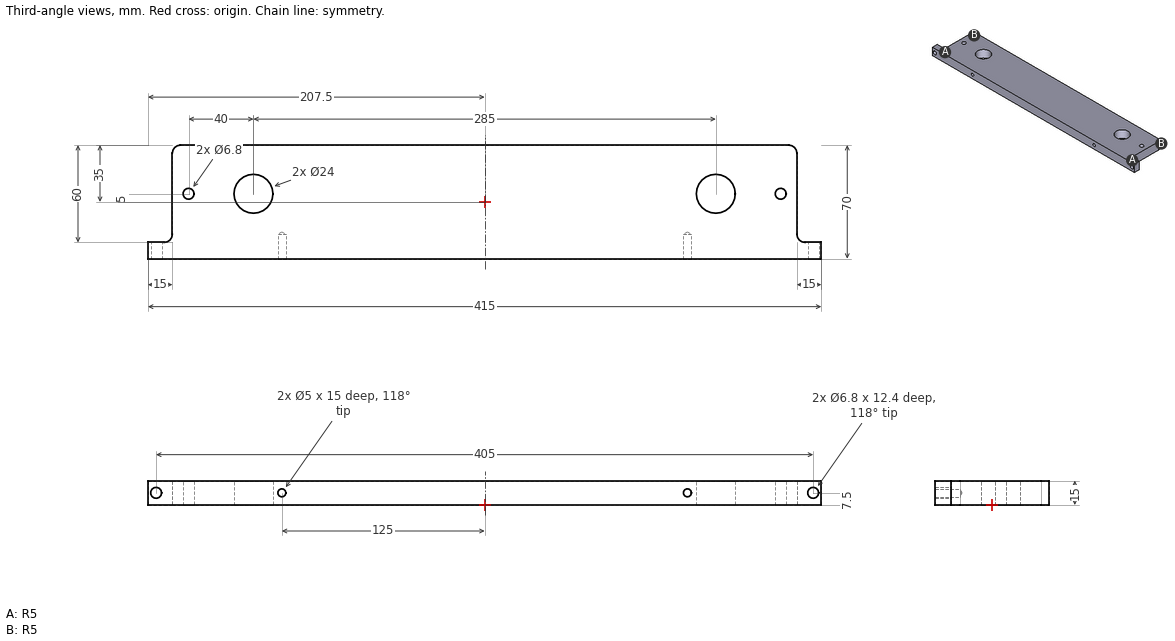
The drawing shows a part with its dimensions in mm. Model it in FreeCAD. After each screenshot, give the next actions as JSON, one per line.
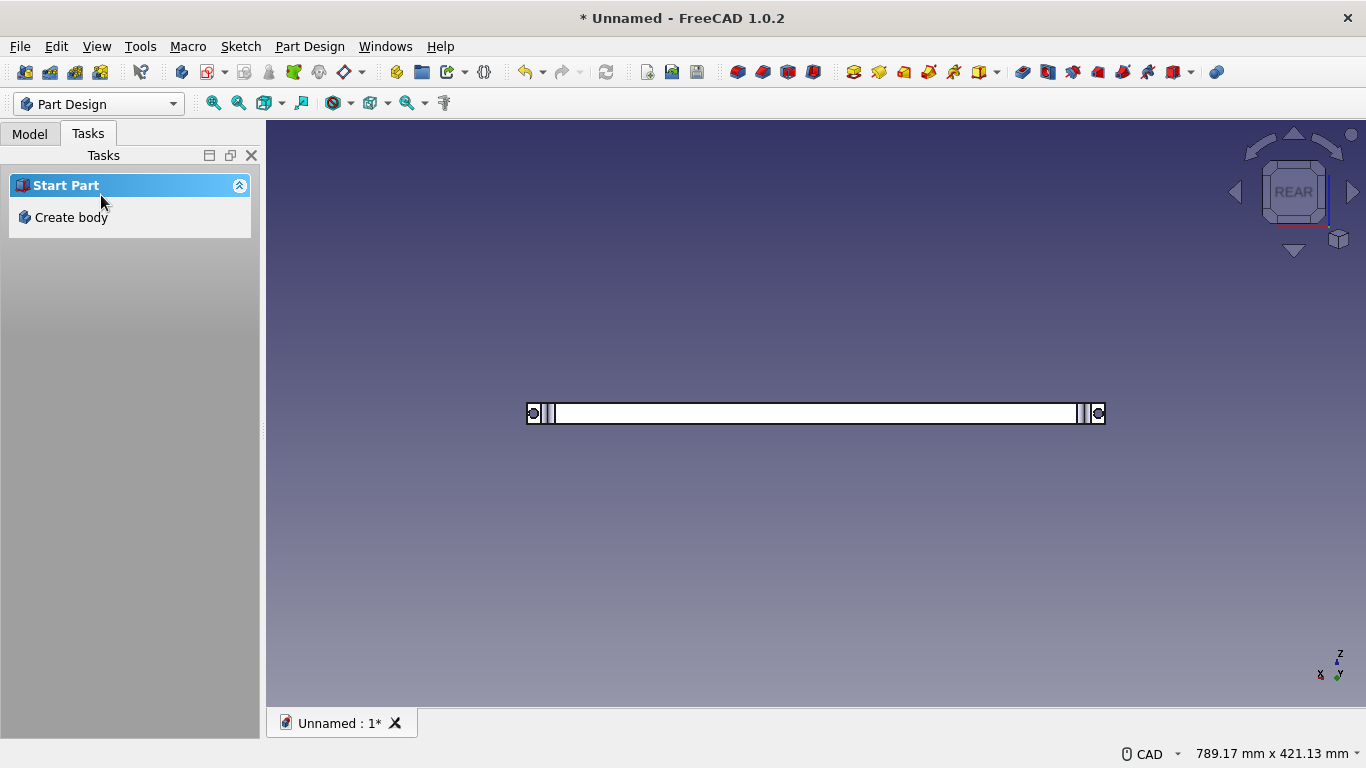
{"action": "key", "text": "0"}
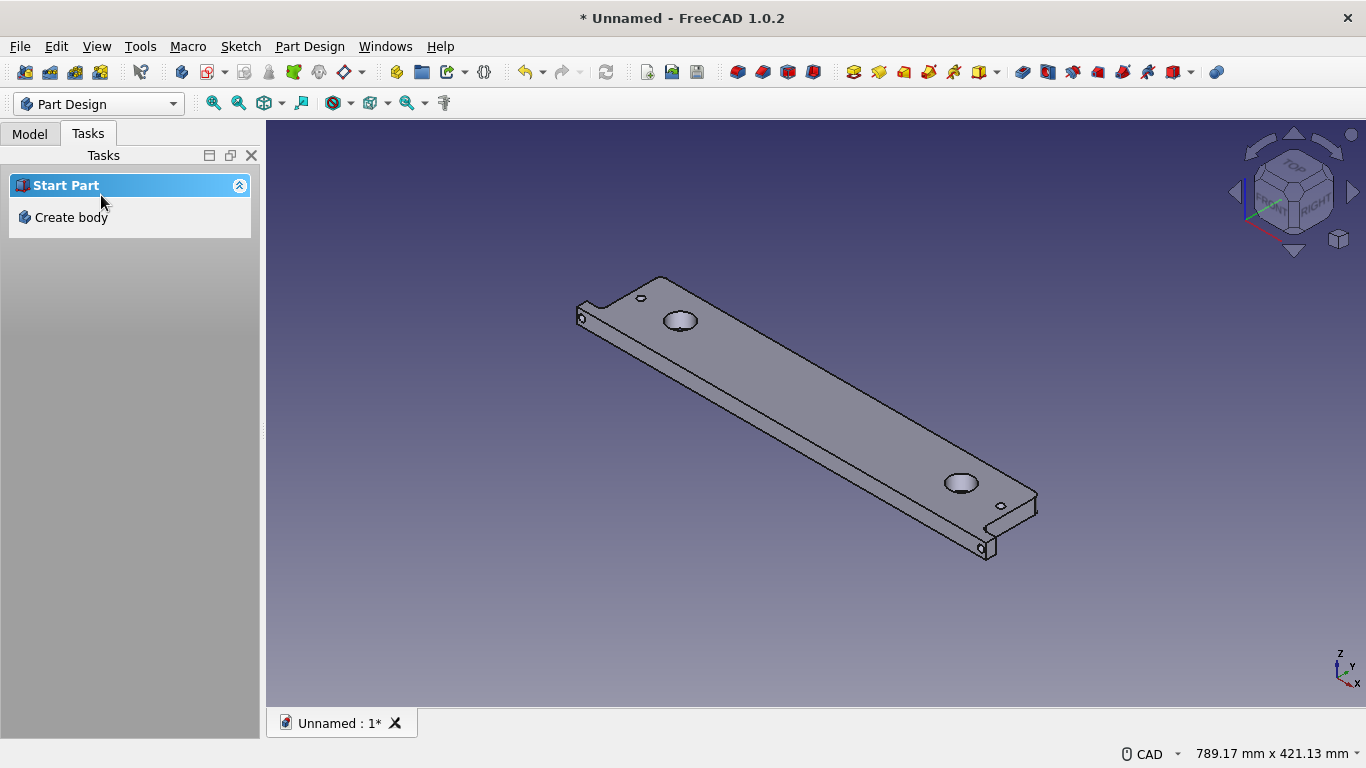
{"action": "key", "text": "1"}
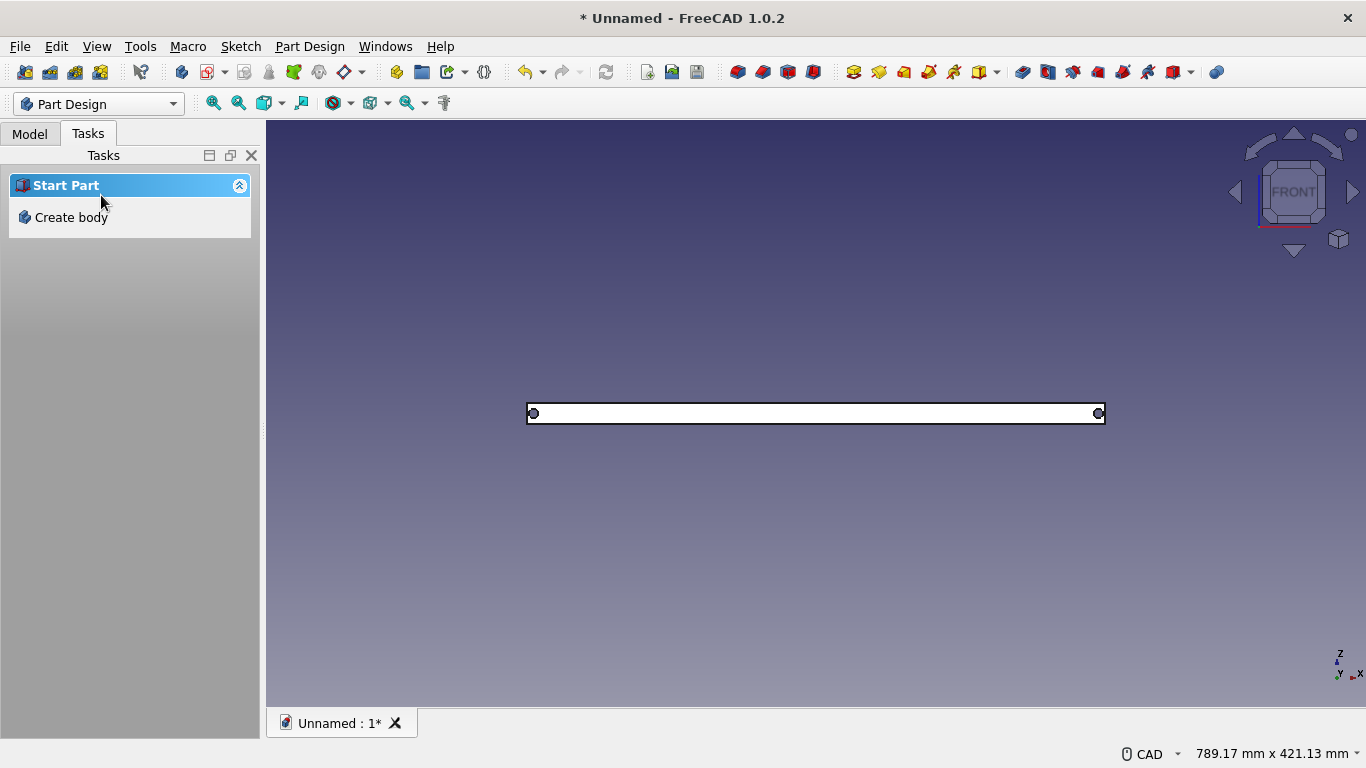
{"action": "left_click", "coordinate": [1064, 412]}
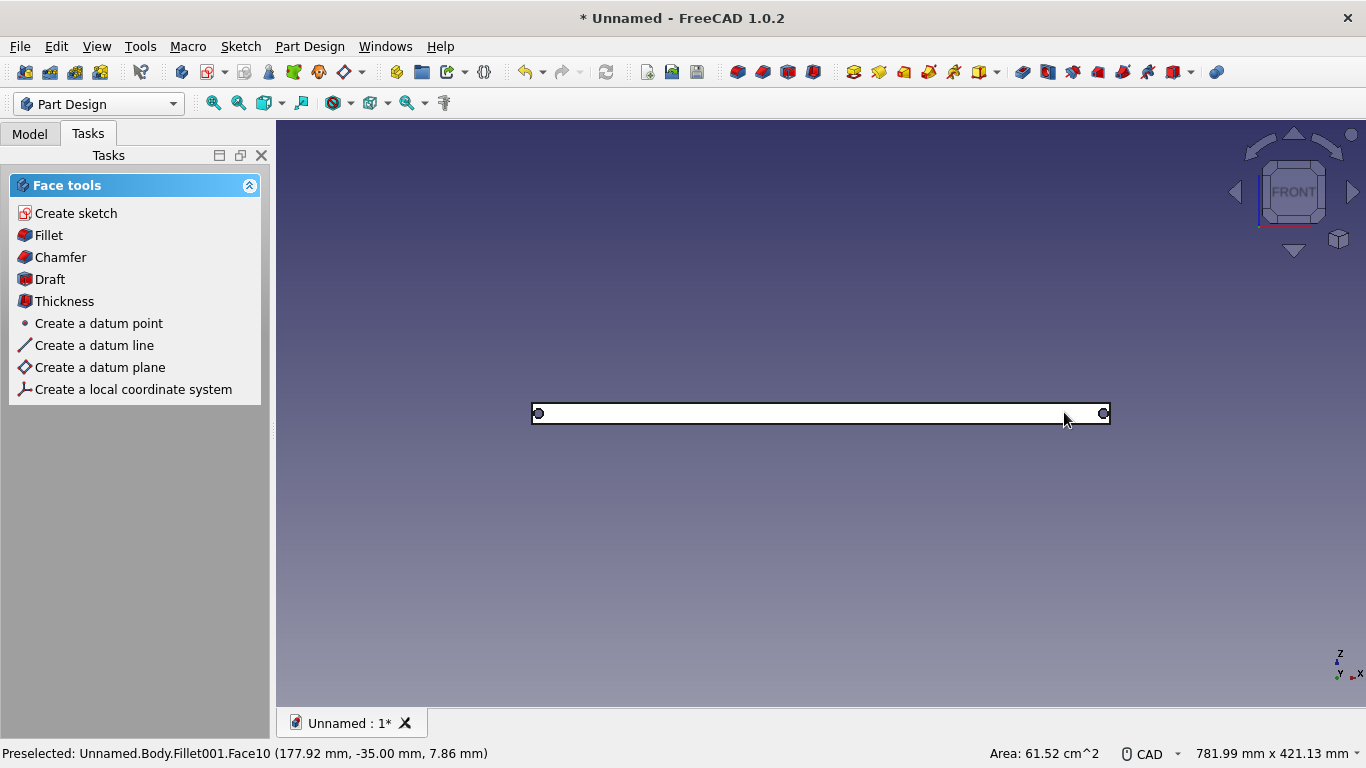
{"action": "left_click", "coordinate": [206, 72]}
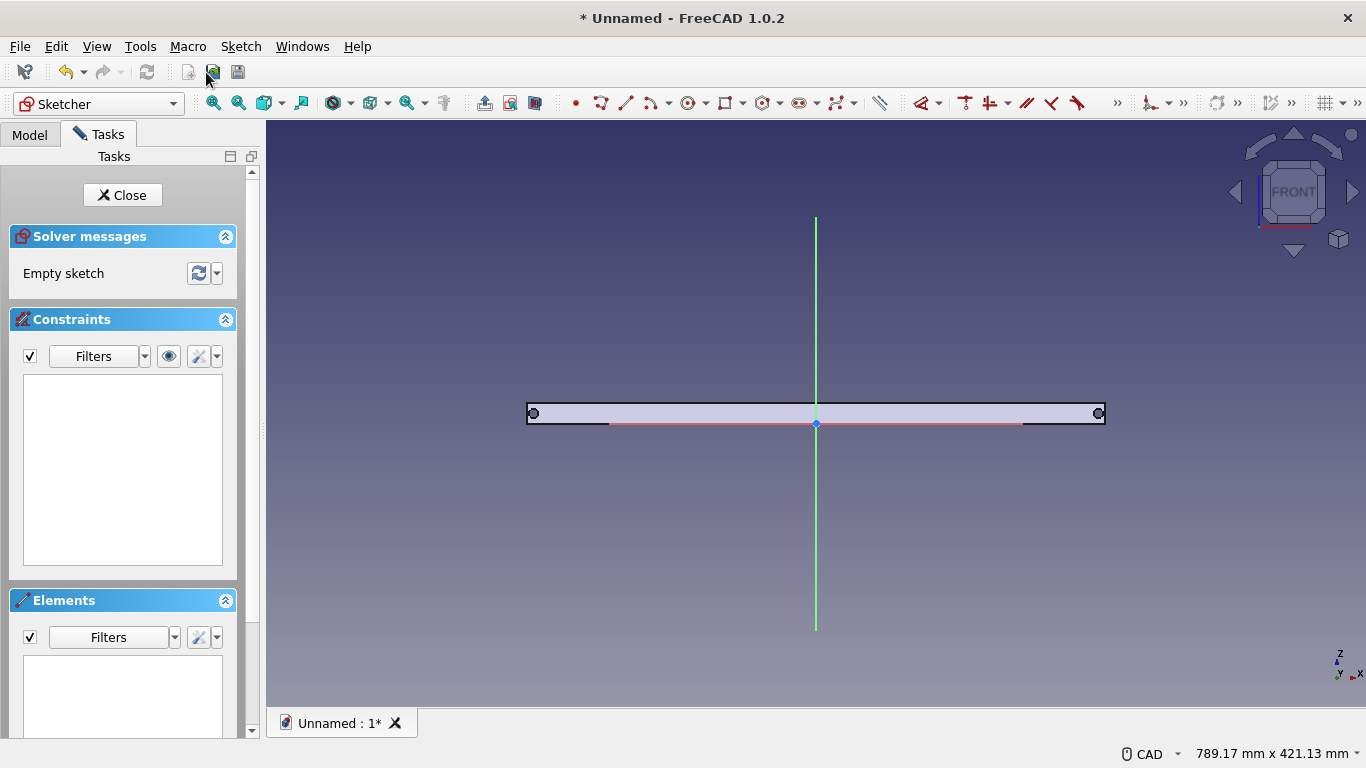
{"action": "scroll", "coordinate": [899, 421], "scroll_direction": "up", "scroll_amount": 3}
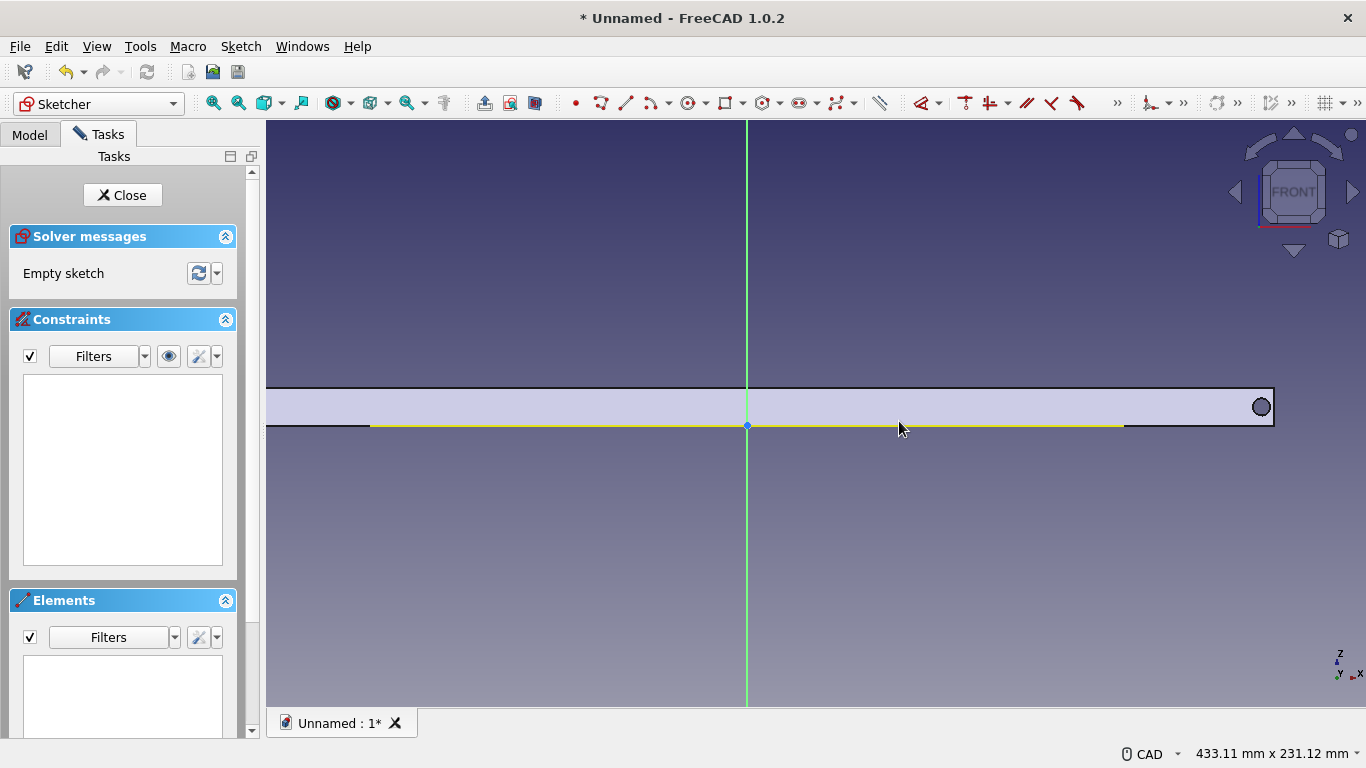
{"action": "key", "text": "g c"}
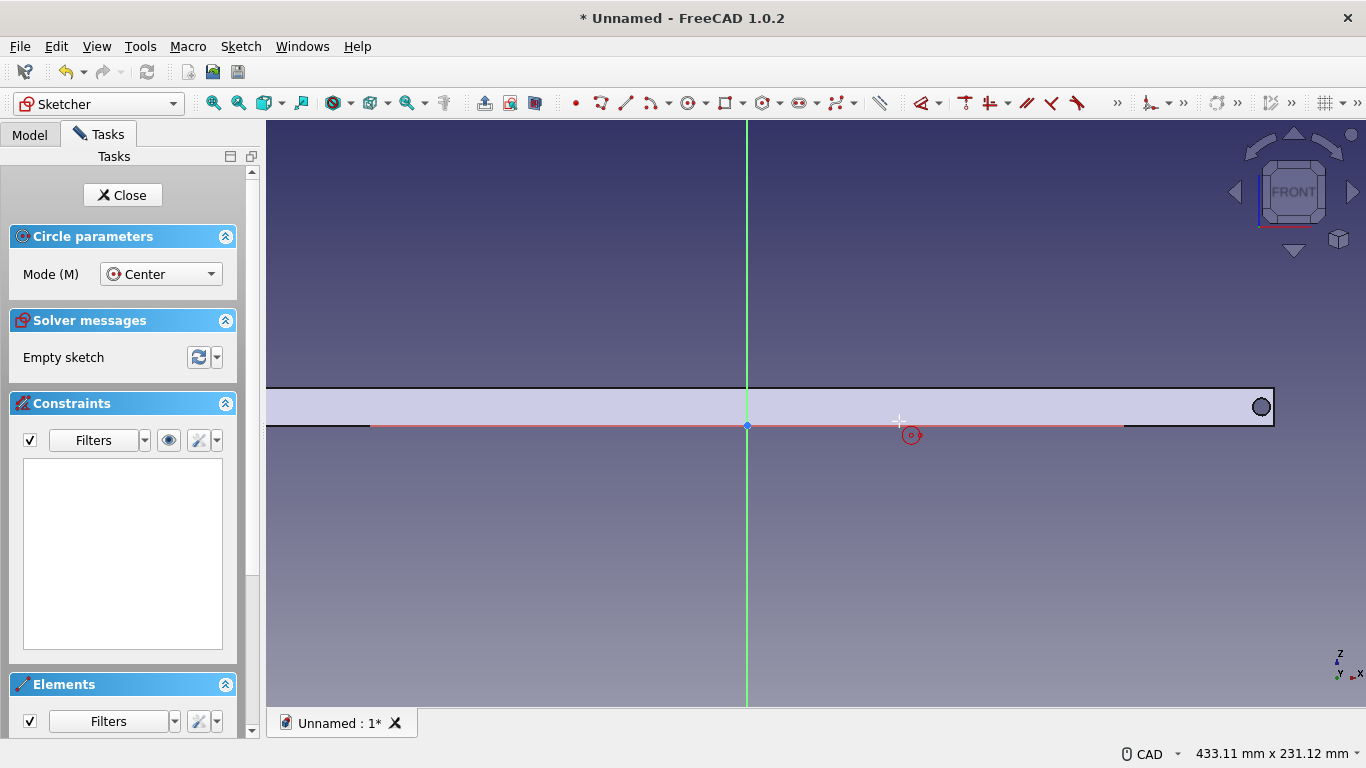
{"action": "scroll", "coordinate": [430, 407], "scroll_direction": "up", "scroll_amount": 7}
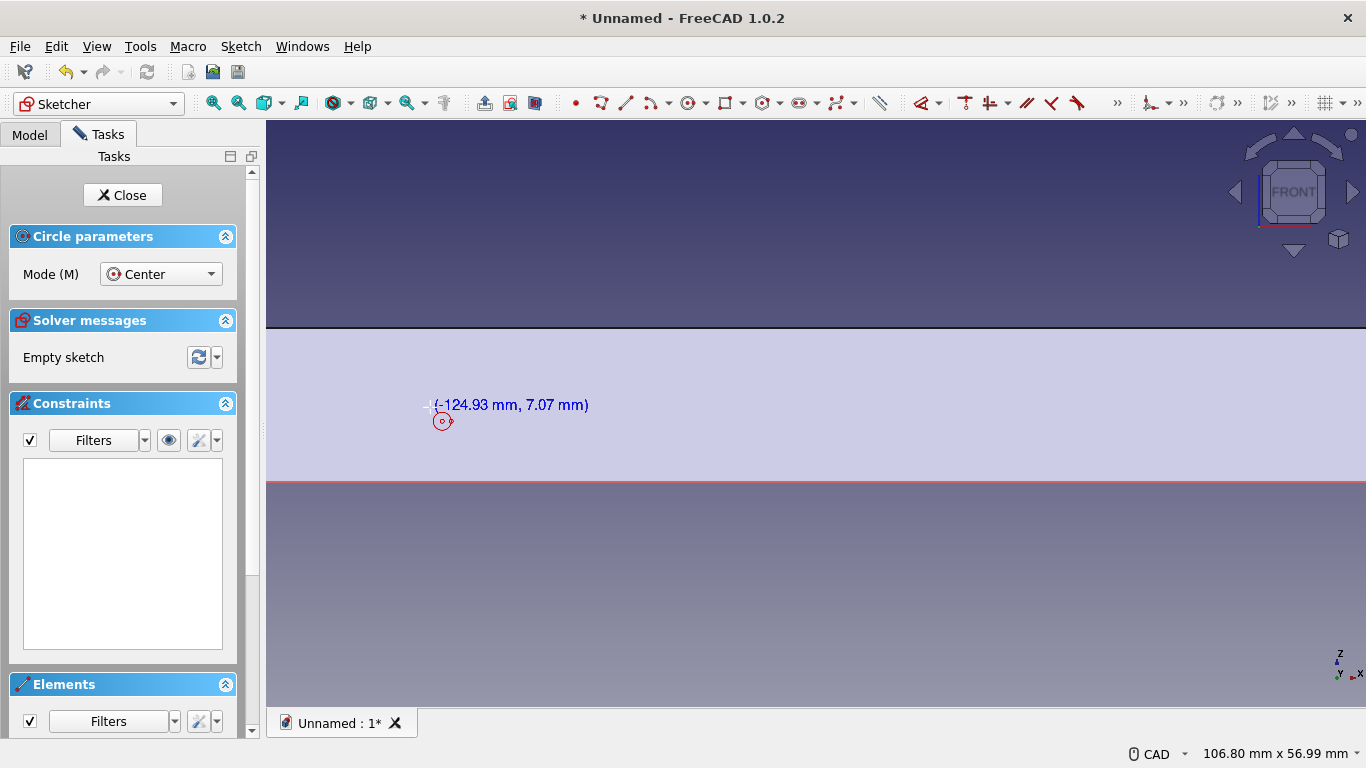
{"action": "scroll", "coordinate": [430, 408], "scroll_direction": "down", "scroll_amount": 7}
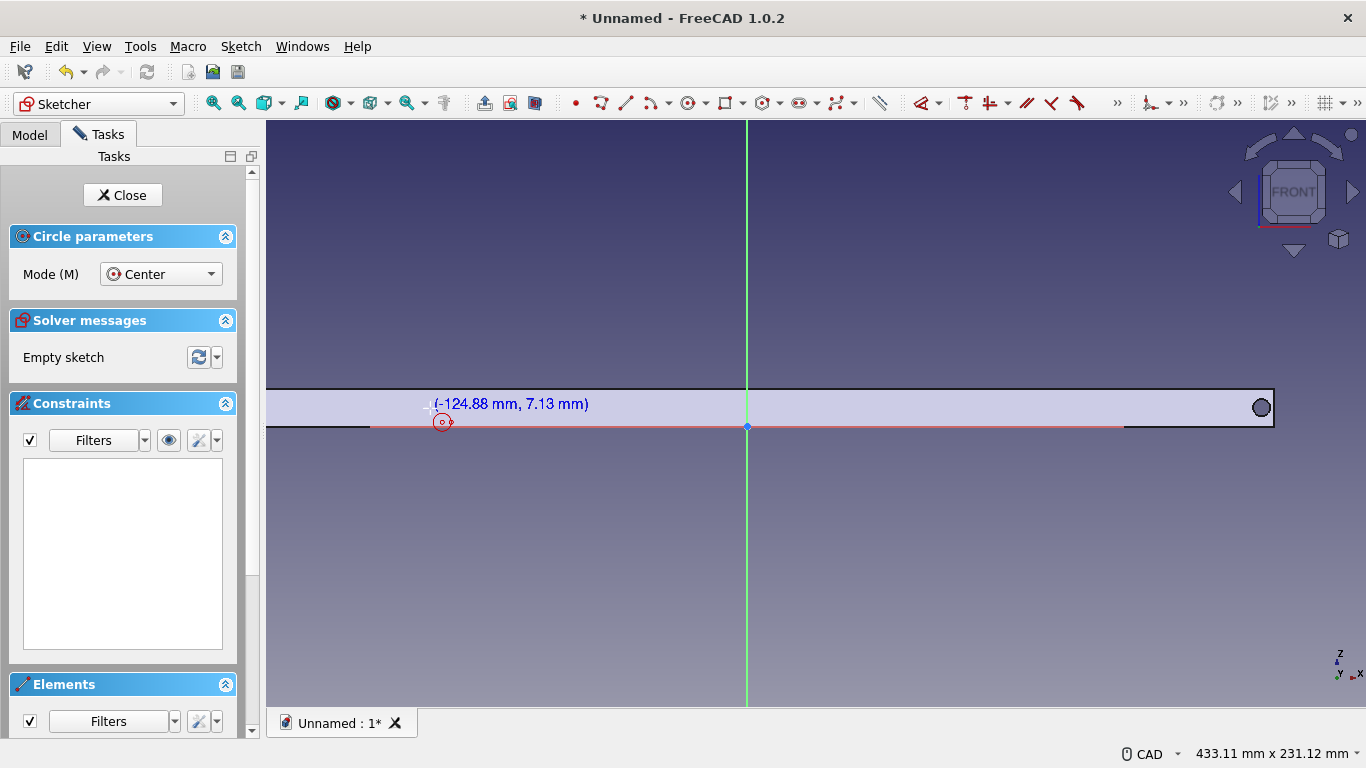
{"action": "left_click", "coordinate": [430, 408]}
{"action": "mouse_move", "coordinate": [434, 403]}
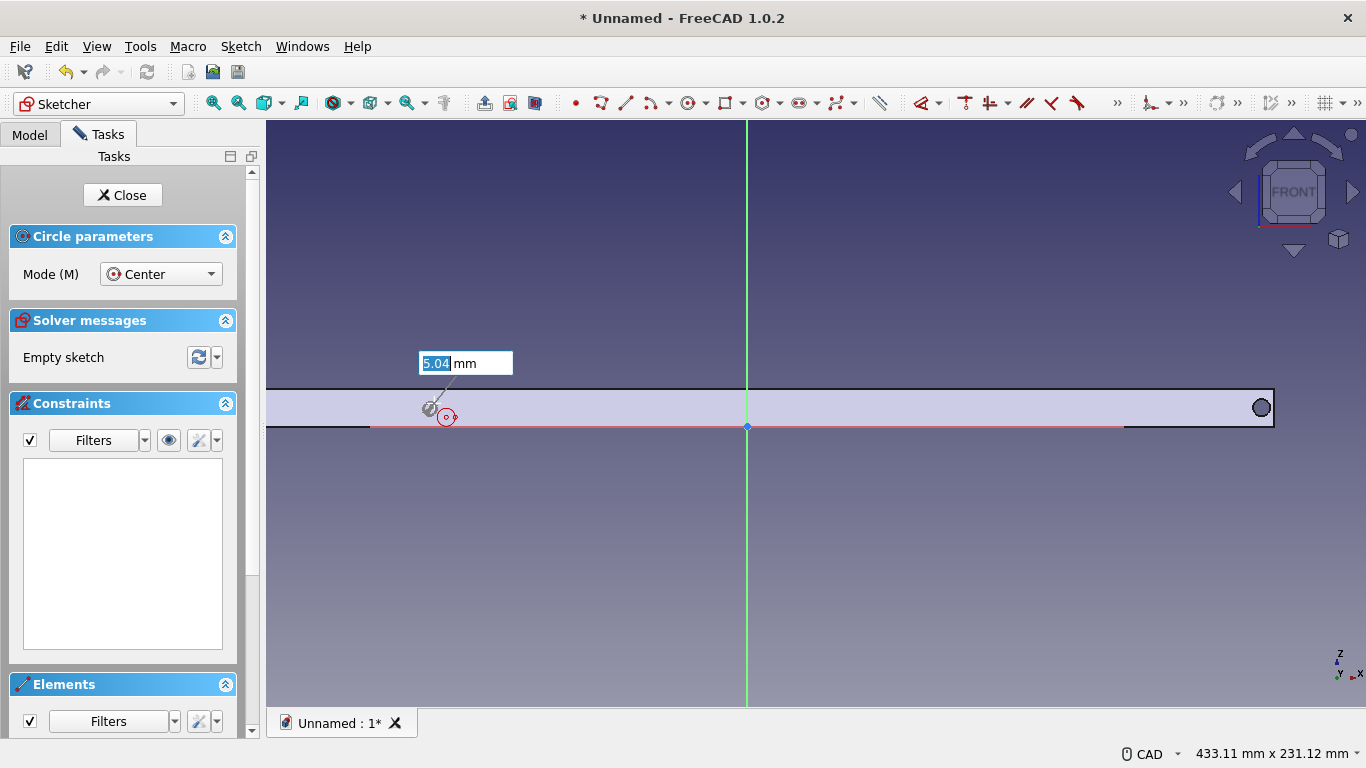
{"action": "type", "text": "5"}
{"action": "key", "text": "Return"}